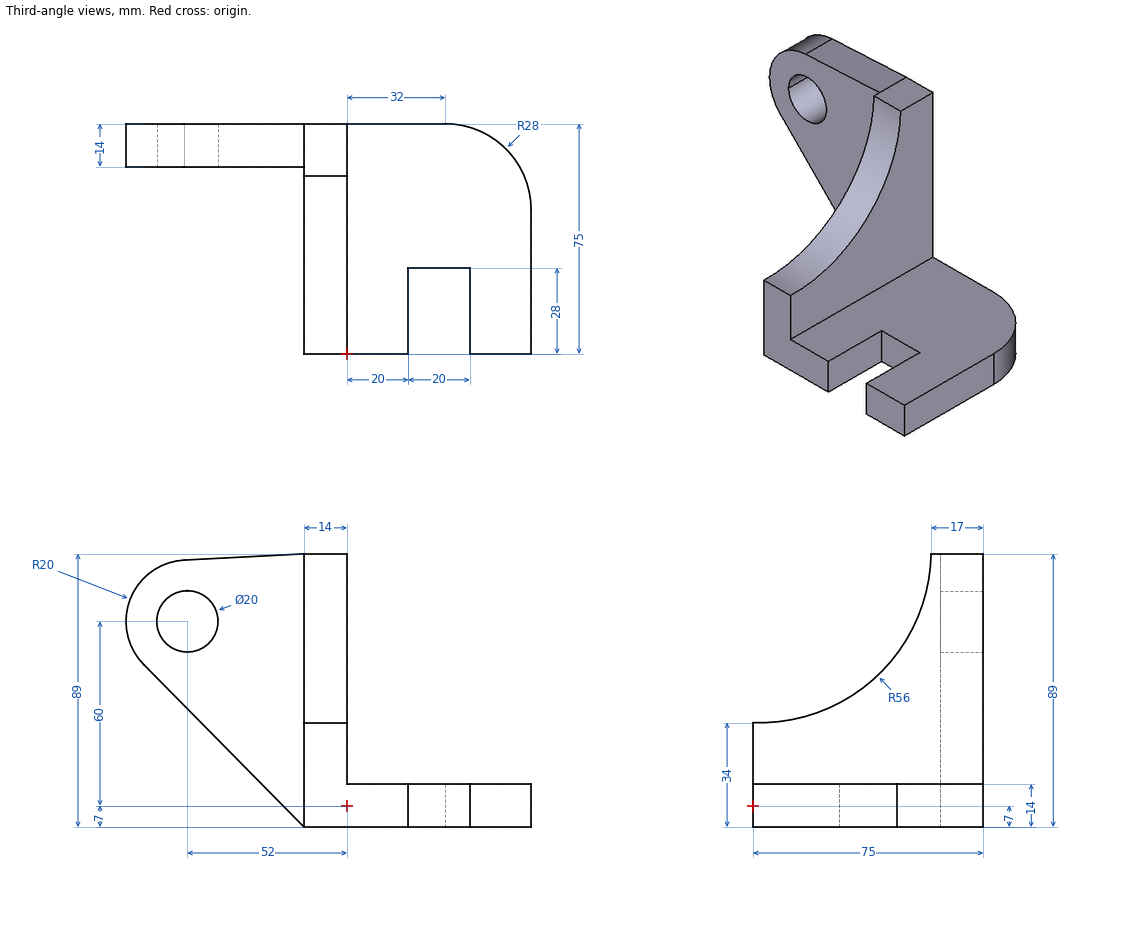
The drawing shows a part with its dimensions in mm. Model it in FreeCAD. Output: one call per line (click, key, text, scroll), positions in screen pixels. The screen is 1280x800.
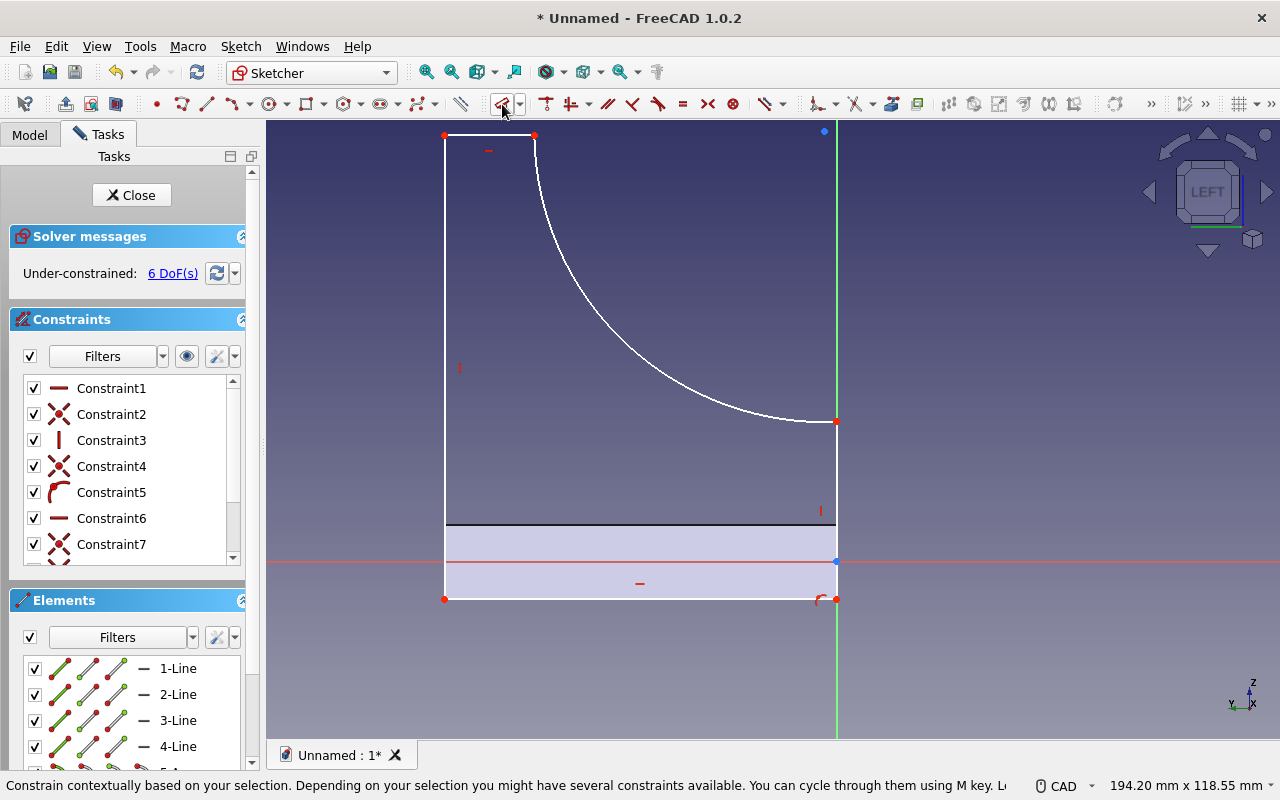
click(569, 269)
click(541, 284)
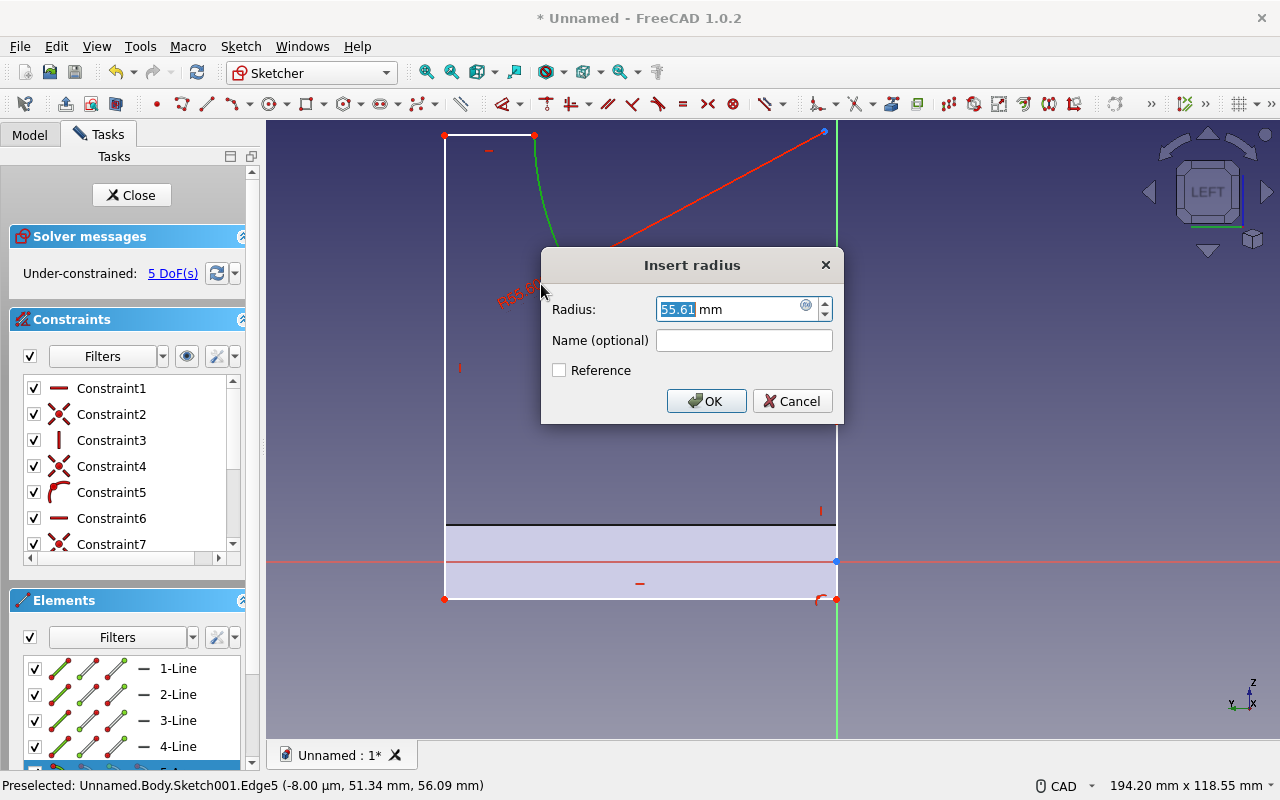
text(56)
key(Return)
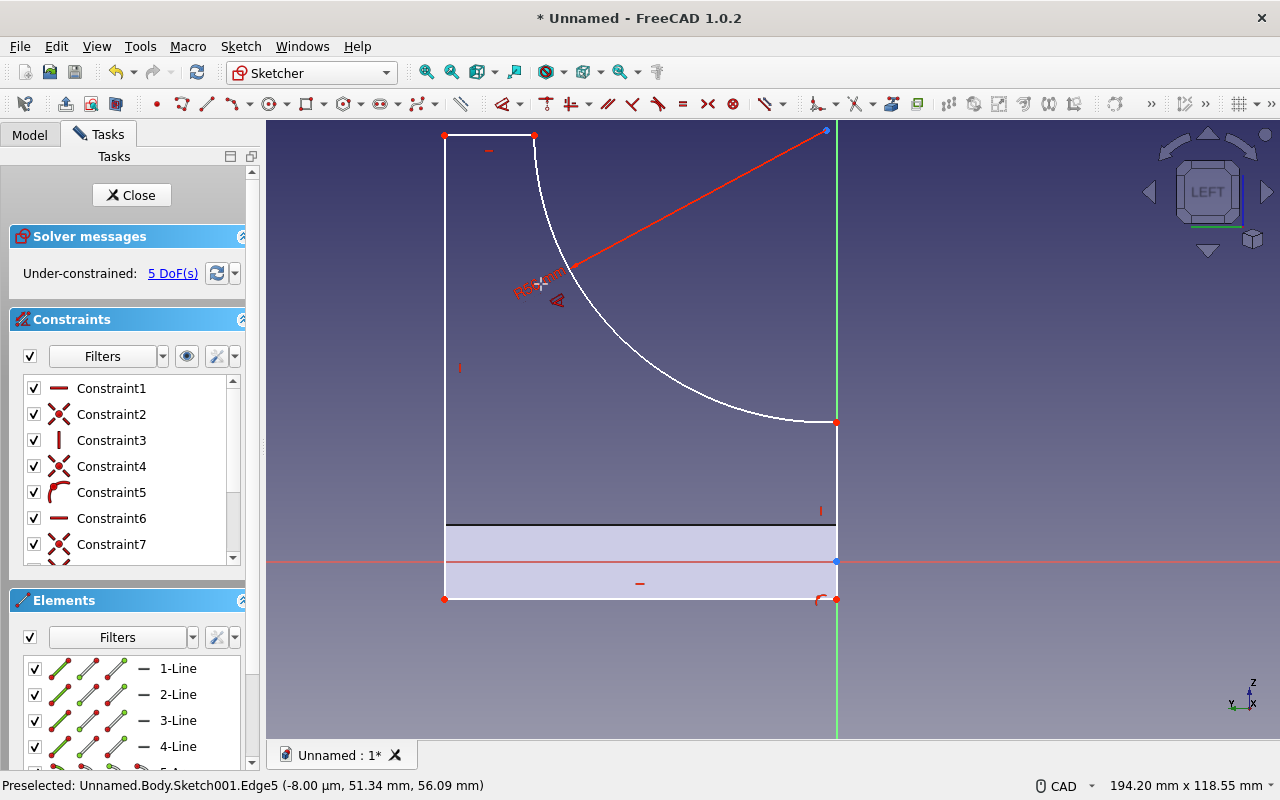
scroll(991, 711, down, 1)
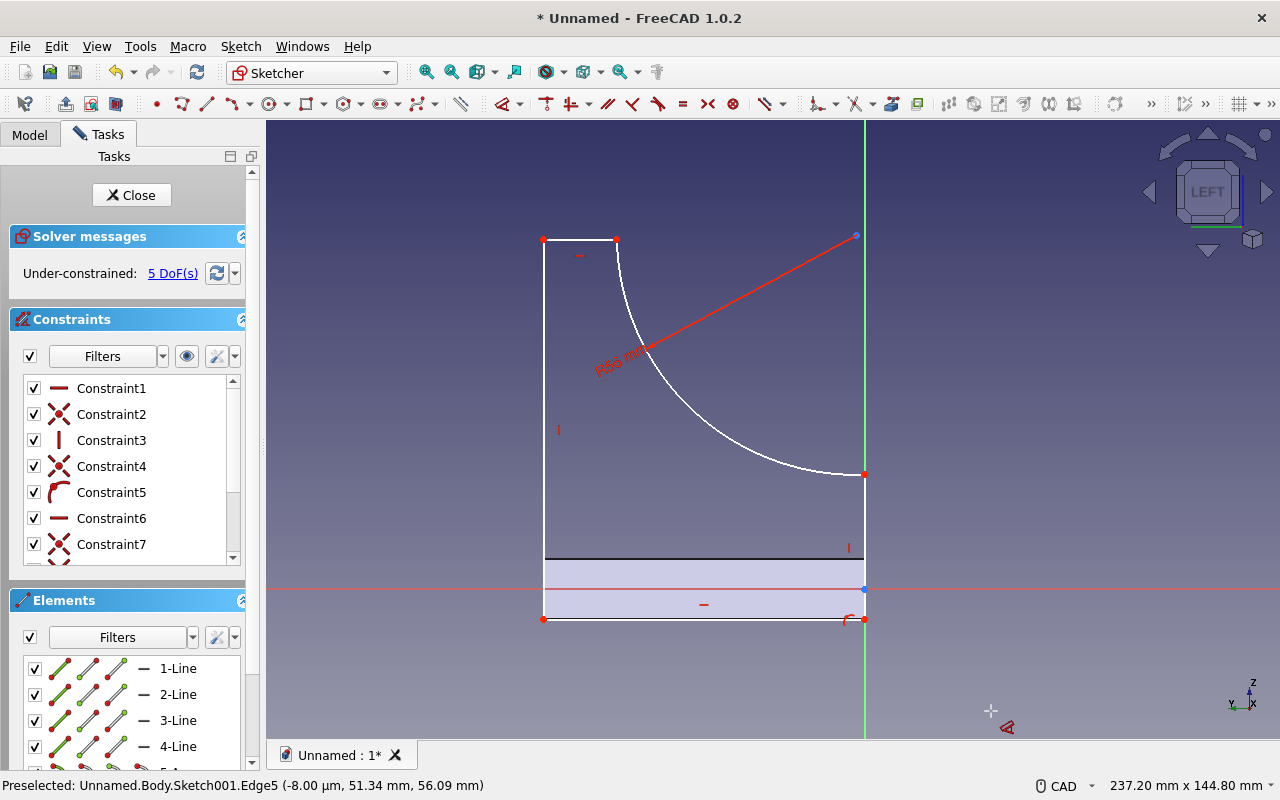
click(595, 240)
click(580, 206)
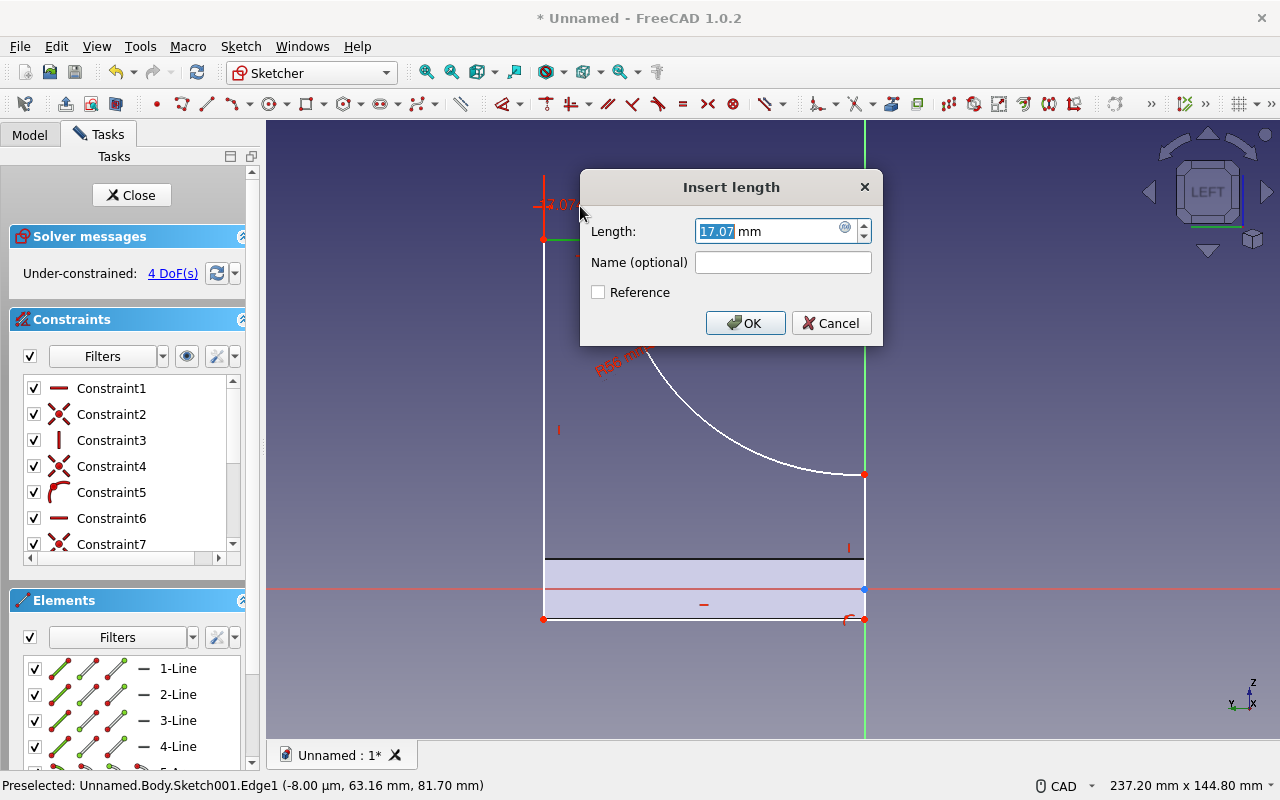
text(17)
key(Return)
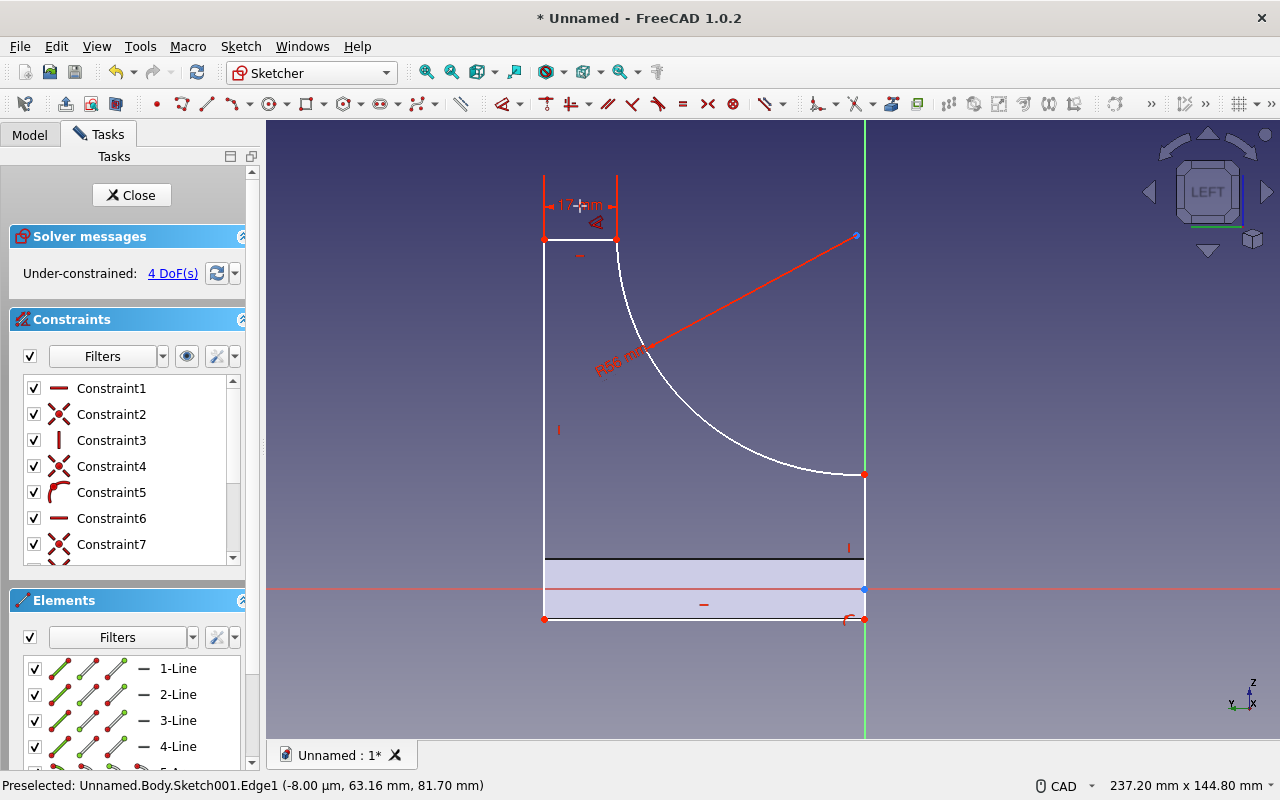
click(544, 354)
click(510, 430)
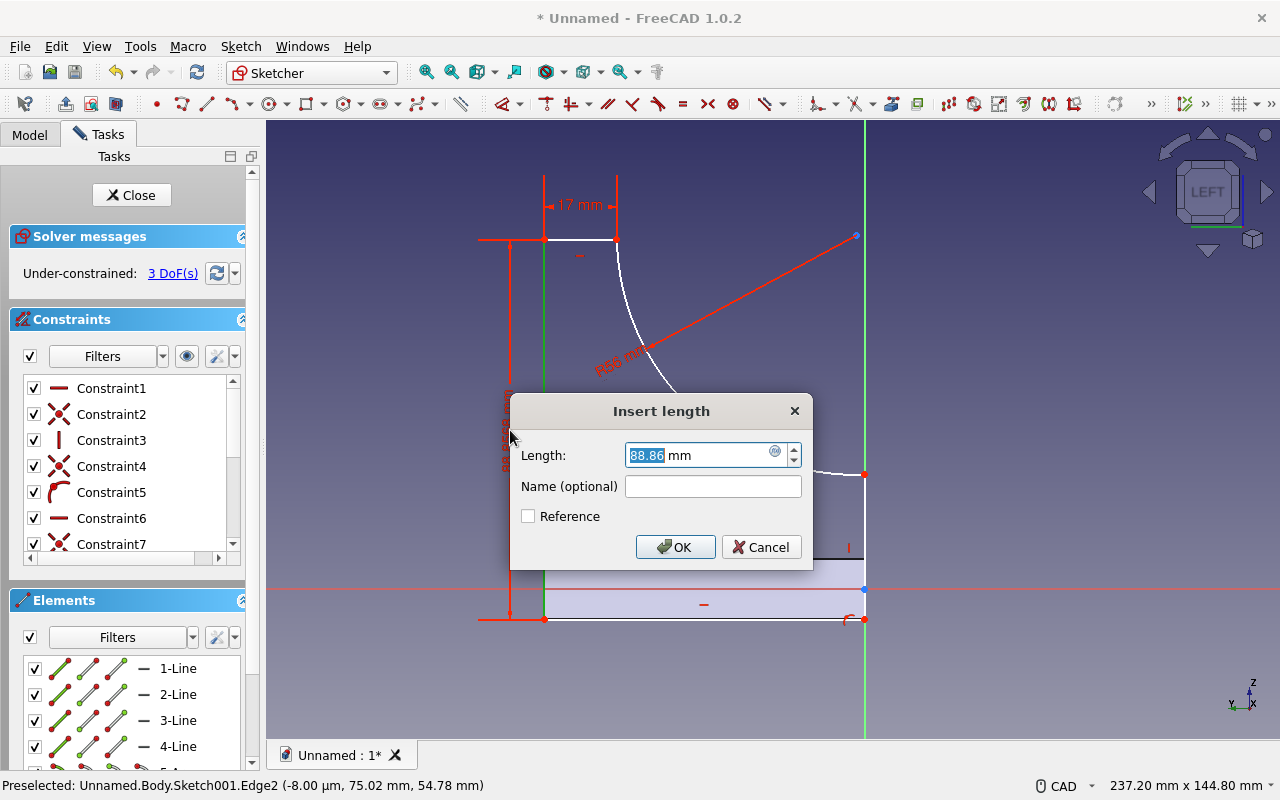
text(89)
key(Return)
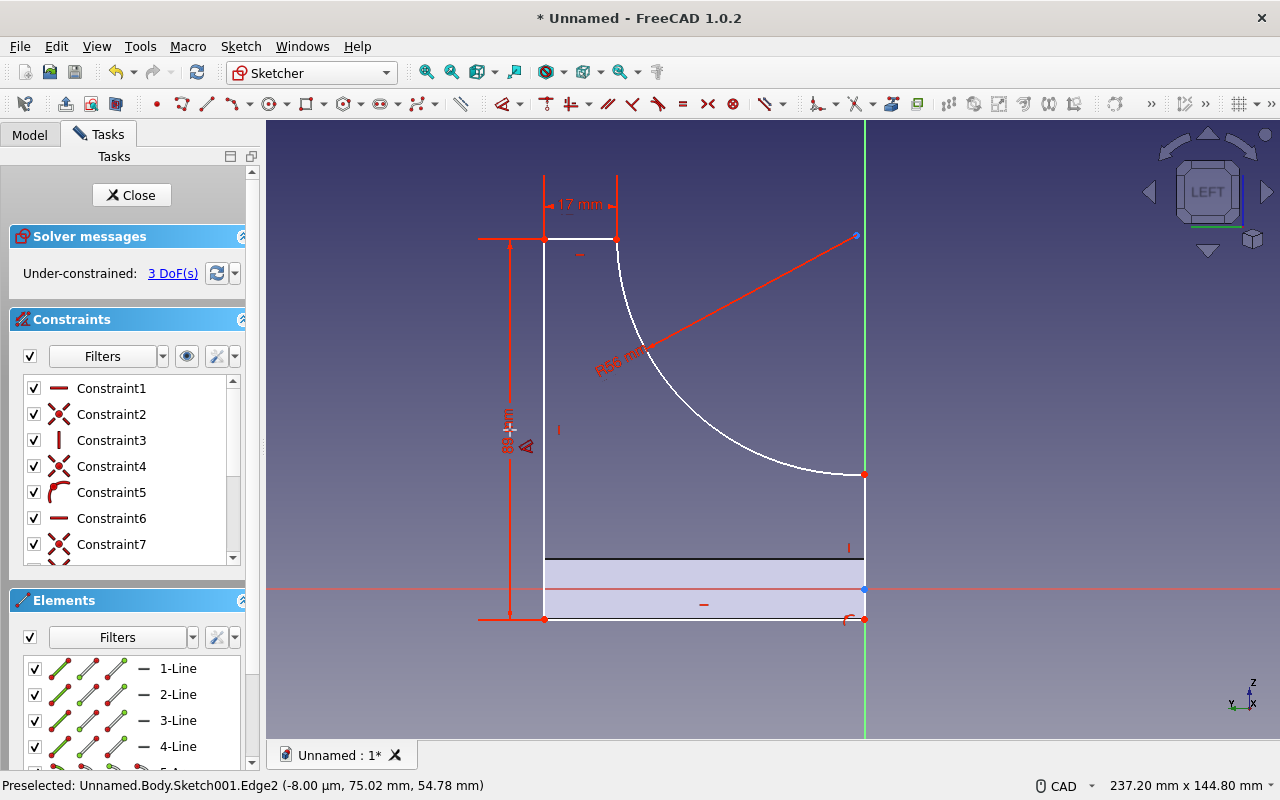
click(641, 620)
click(705, 654)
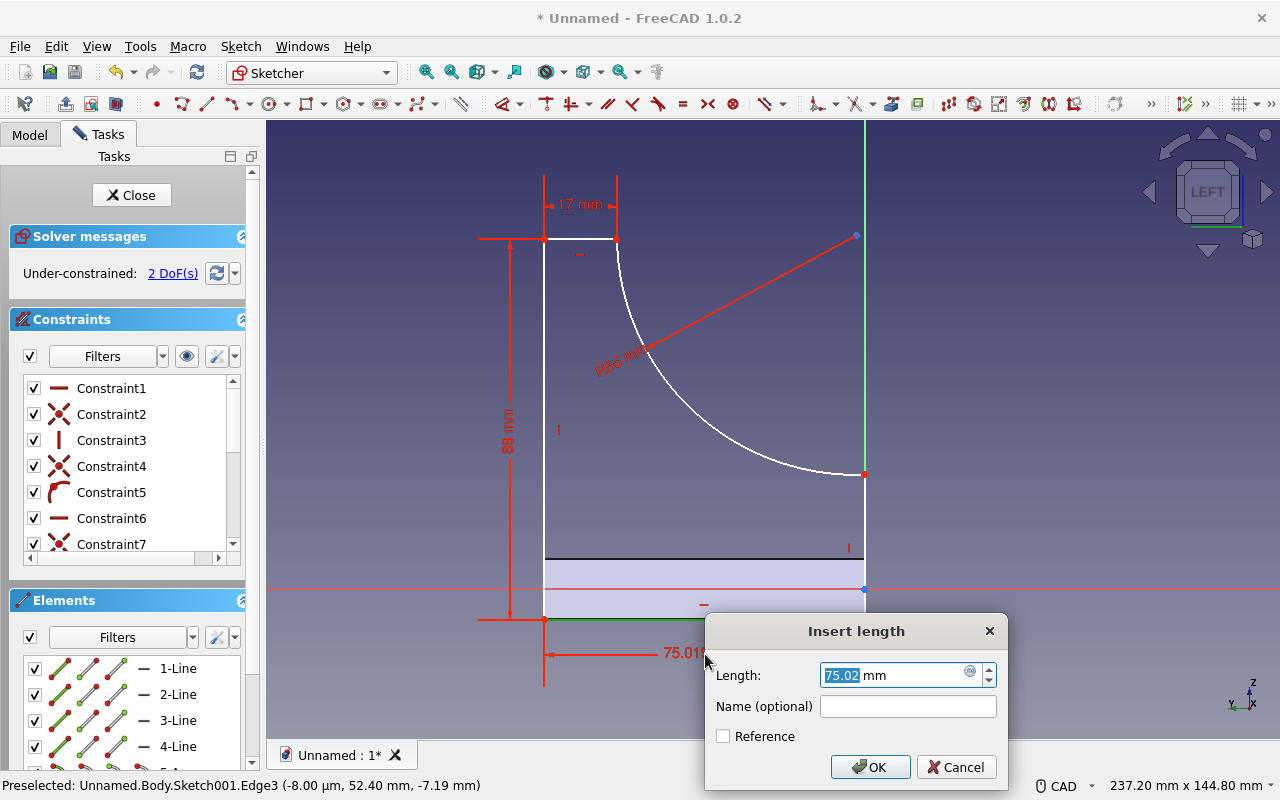
text(75)
key(Return)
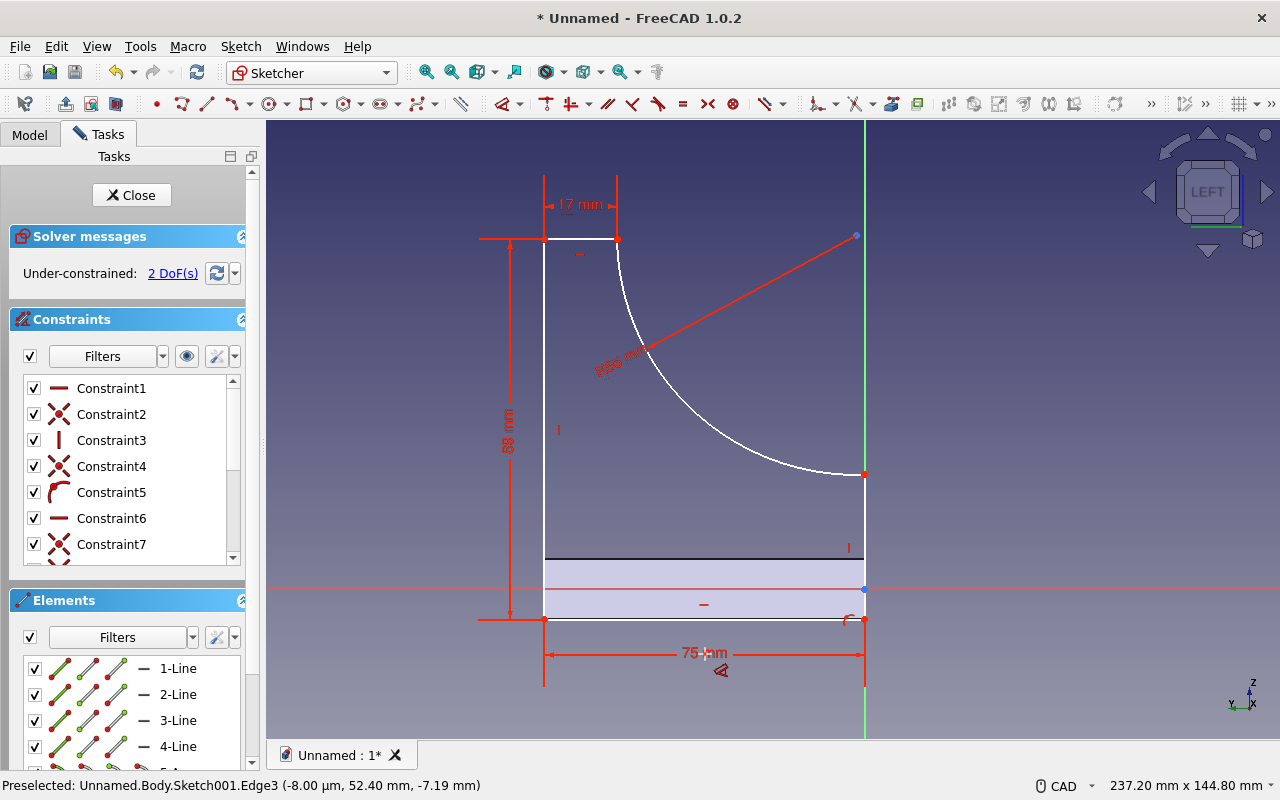
click(865, 576)
click(899, 547)